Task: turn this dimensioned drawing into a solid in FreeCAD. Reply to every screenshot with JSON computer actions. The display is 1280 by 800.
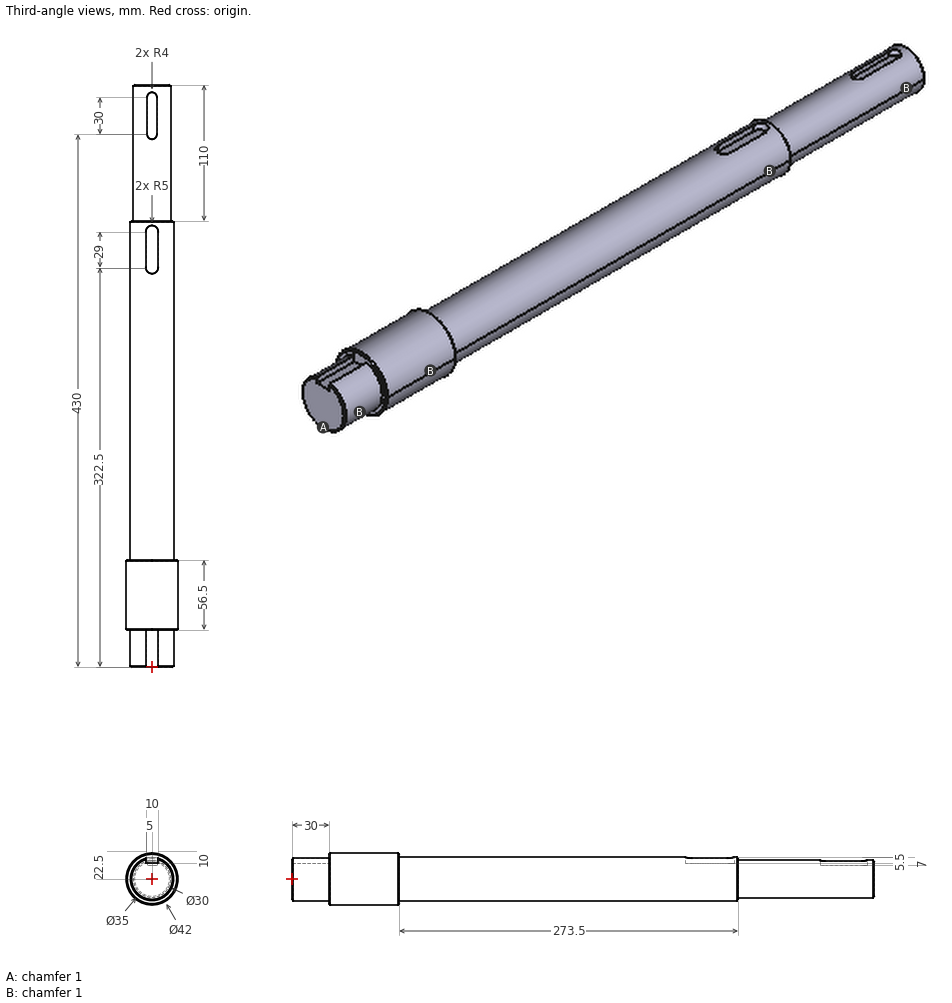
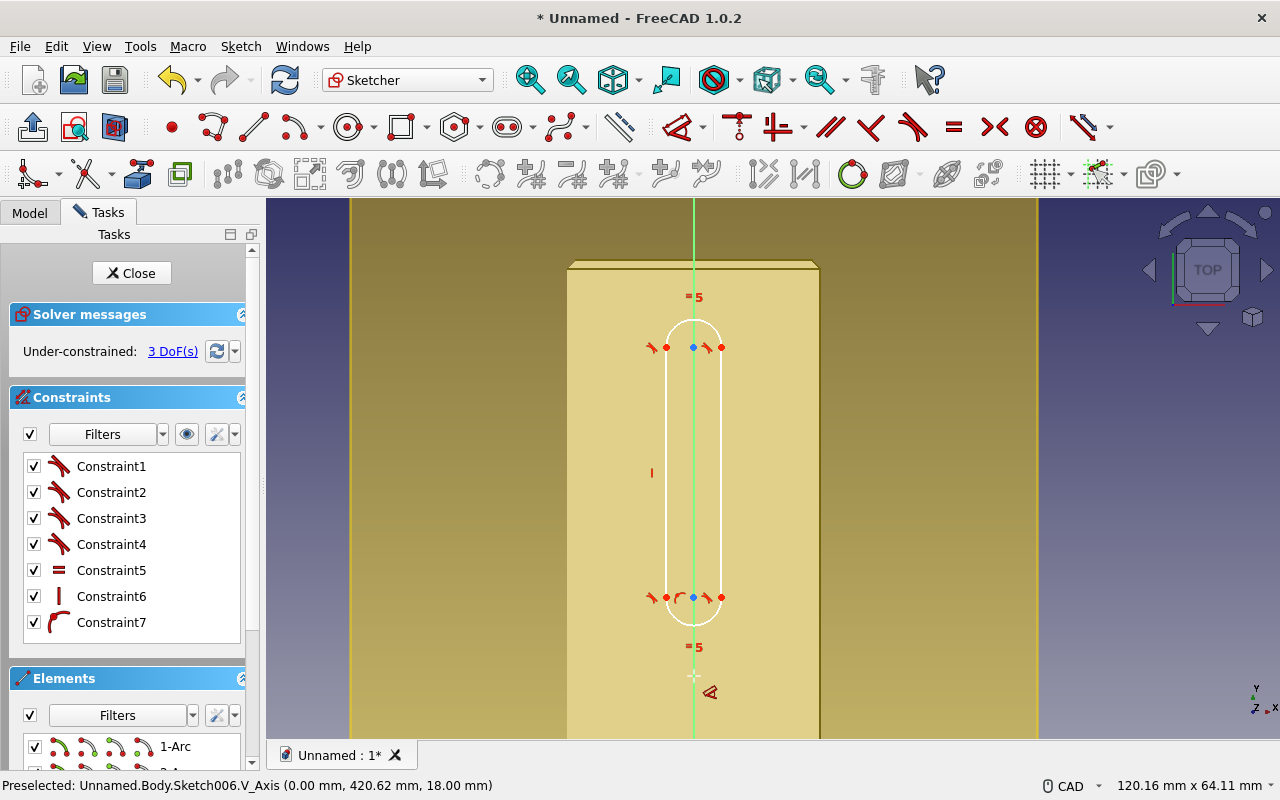
{"action": "left_click", "coordinate": [678, 620]}
{"action": "left_click", "coordinate": [659, 646]}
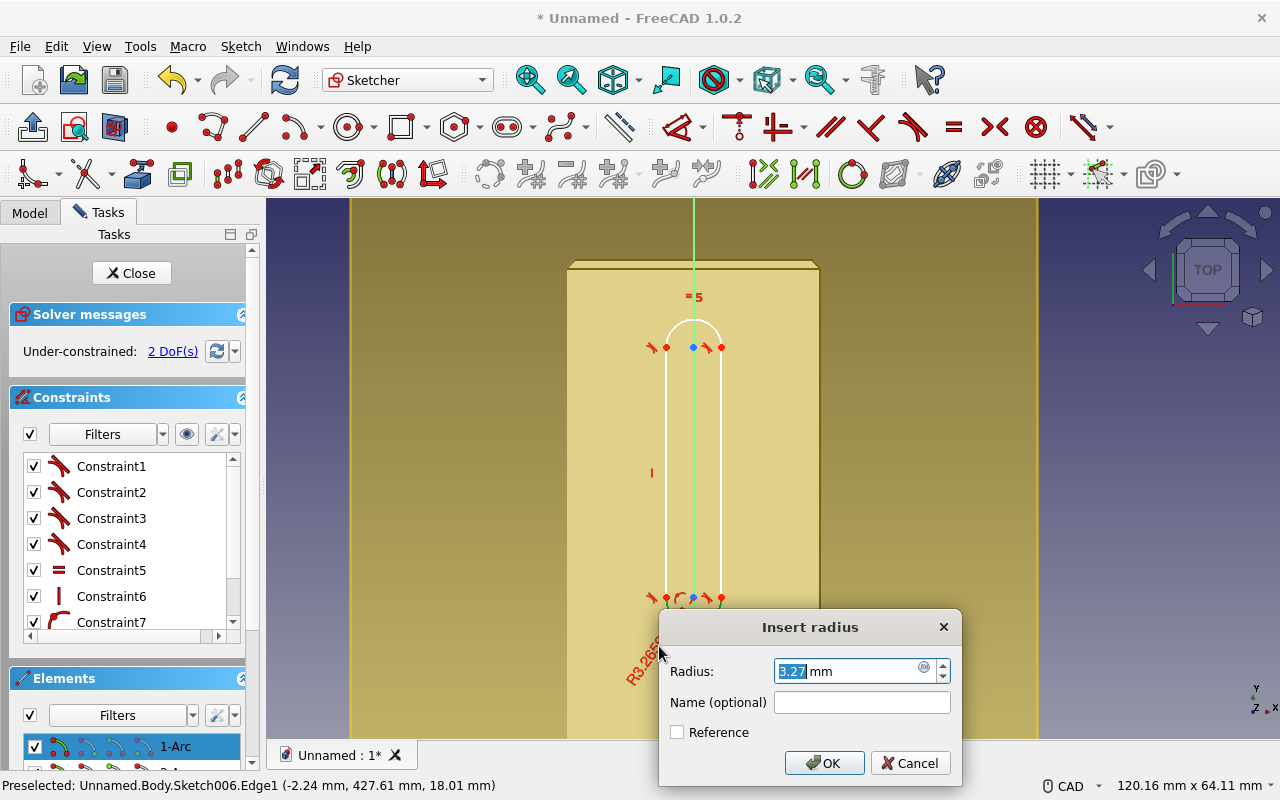
{"action": "type", "text": "4"}
{"action": "key", "text": "Return"}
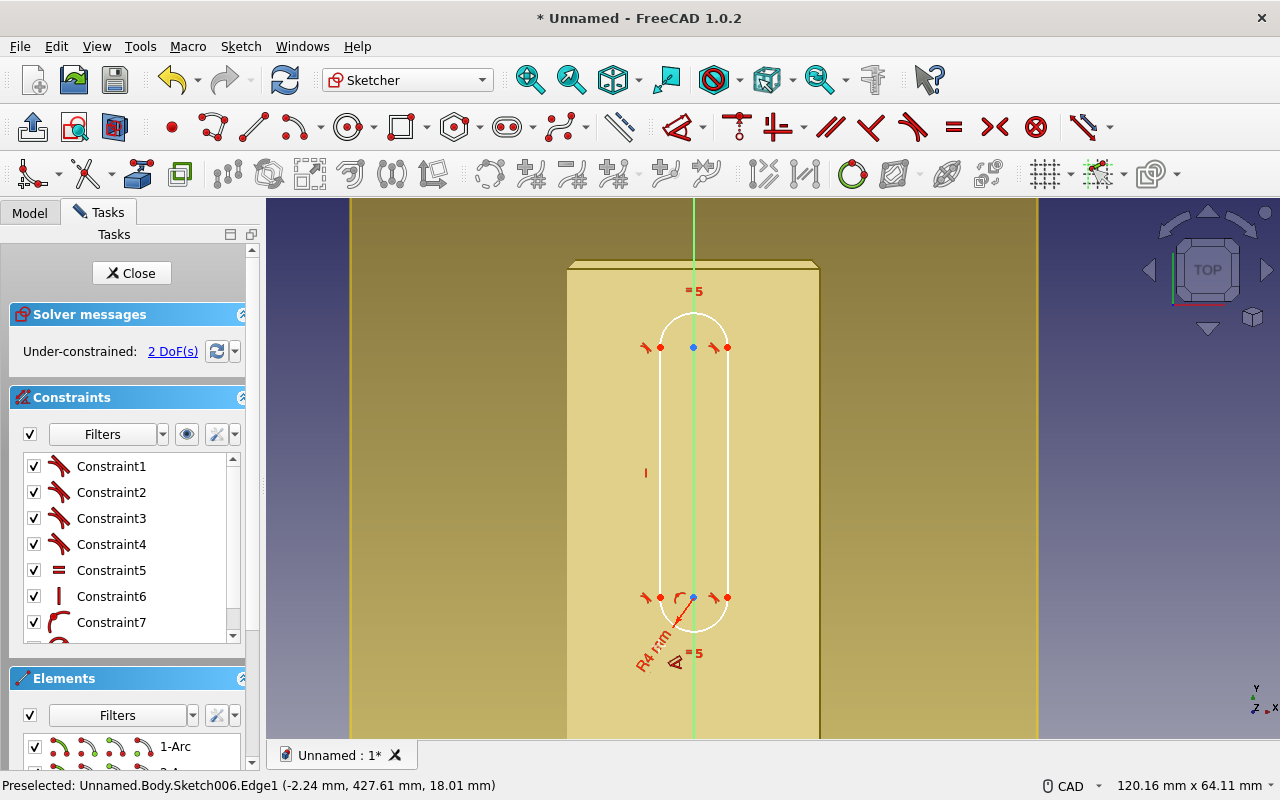
{"action": "left_click", "coordinate": [660, 523]}
{"action": "left_click", "coordinate": [626, 473]}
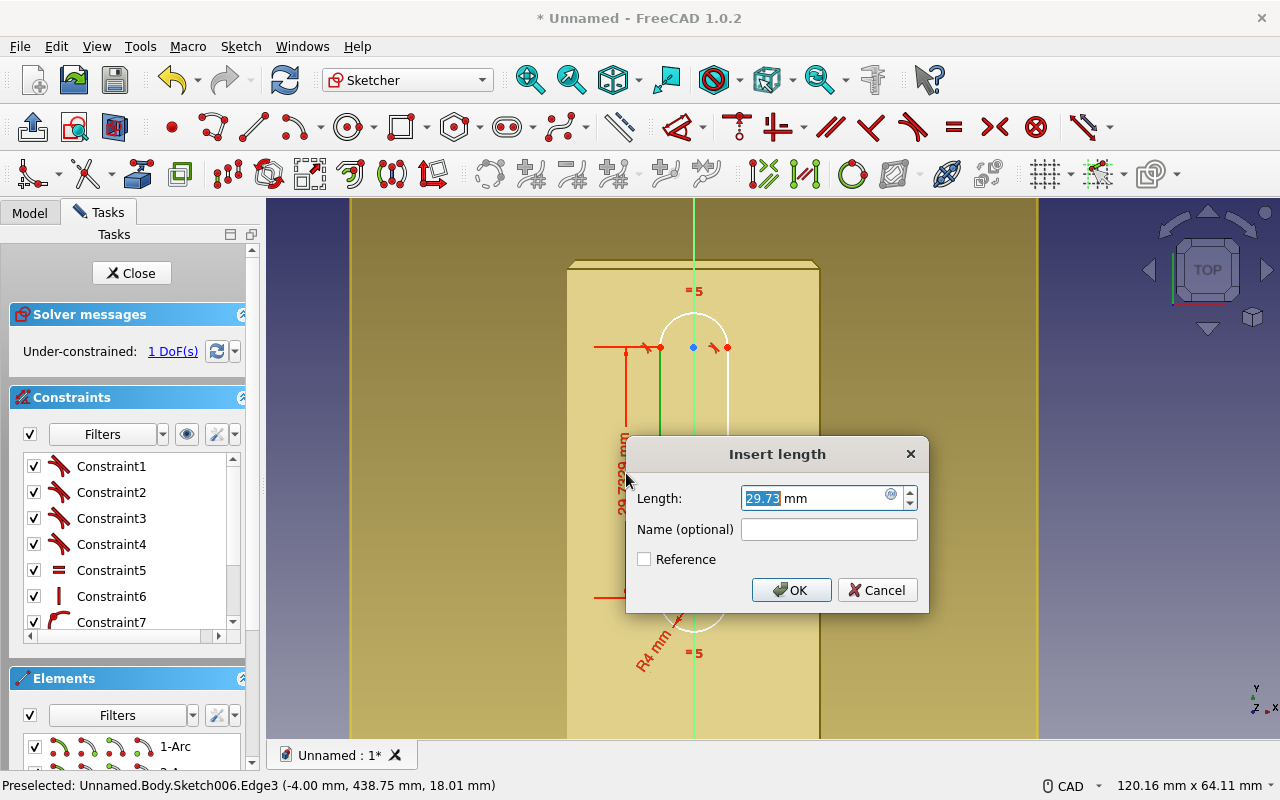
{"action": "type", "text": "30"}
{"action": "key", "text": "Return"}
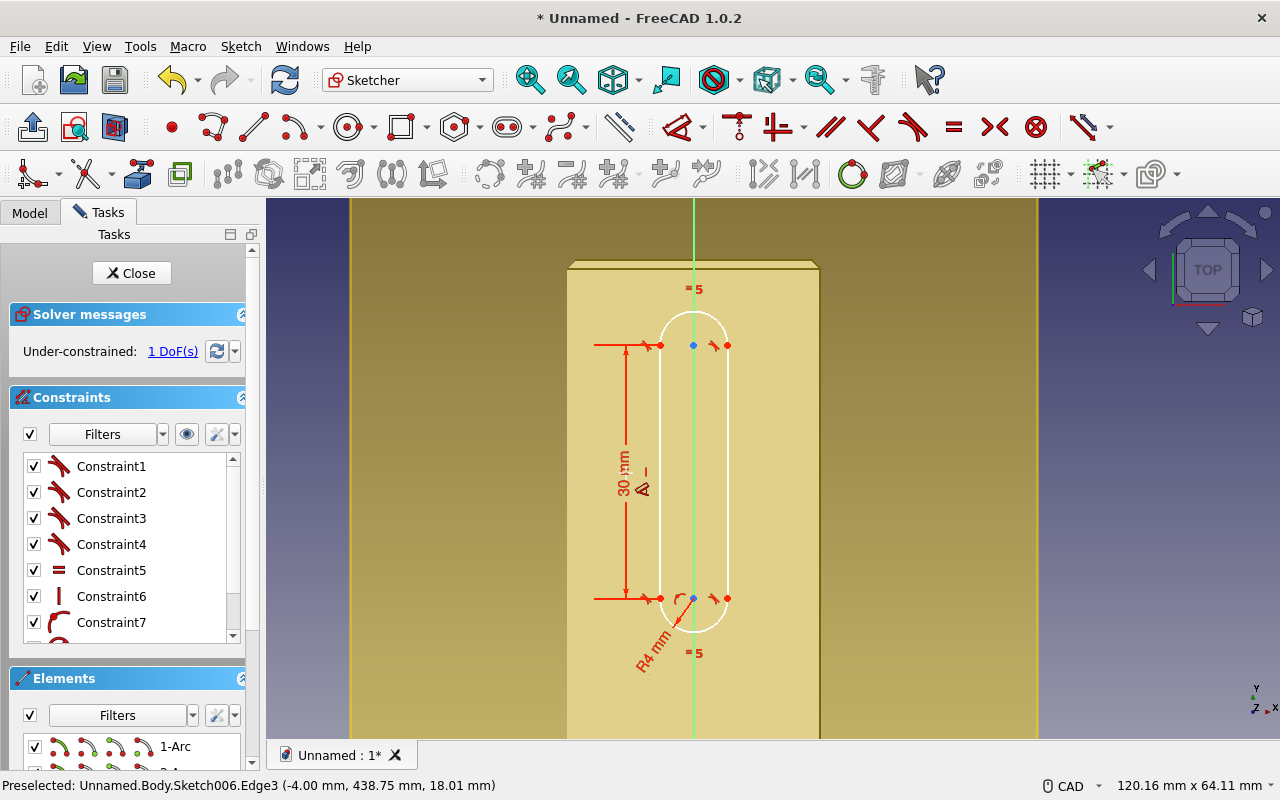
{"action": "left_click", "coordinate": [660, 599]}
{"action": "left_click", "coordinate": [626, 681]}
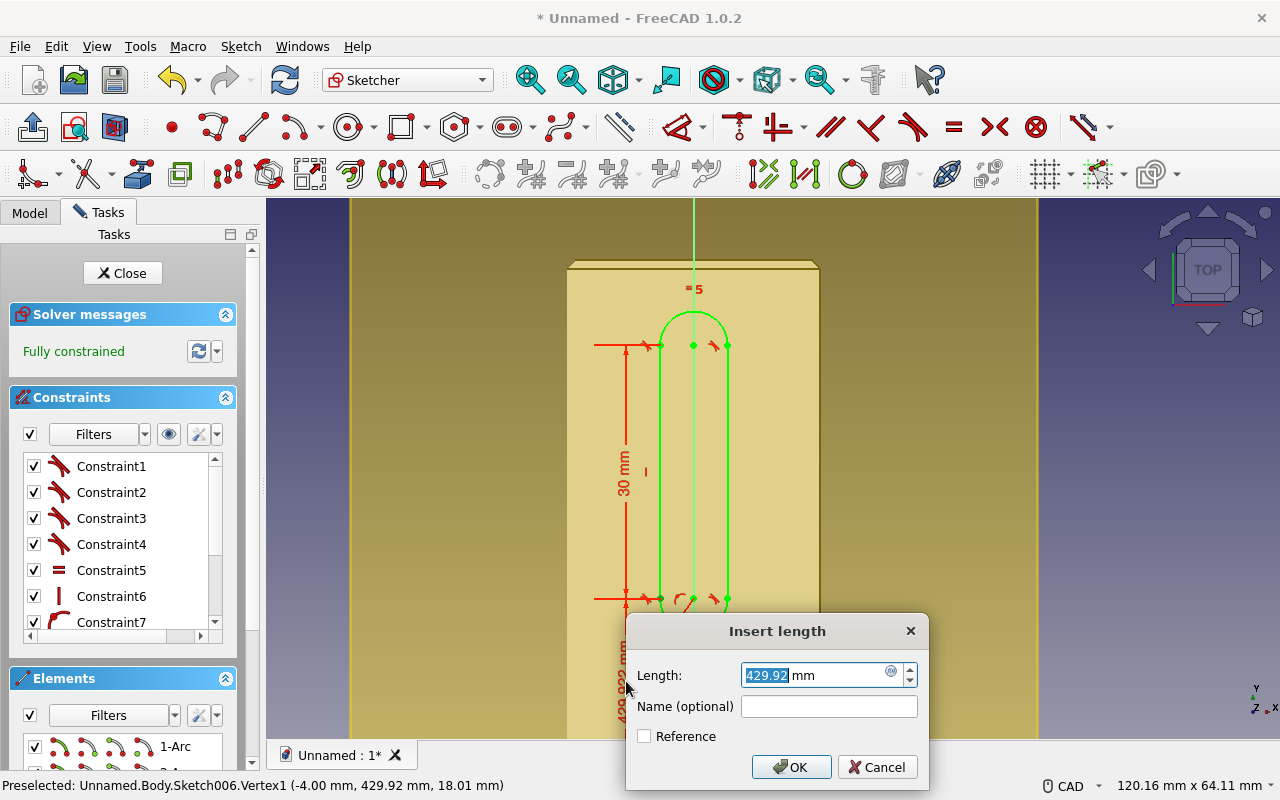
{"action": "type", "text": "430"}
{"action": "key", "text": "Return"}
{"action": "key", "text": "Escape"}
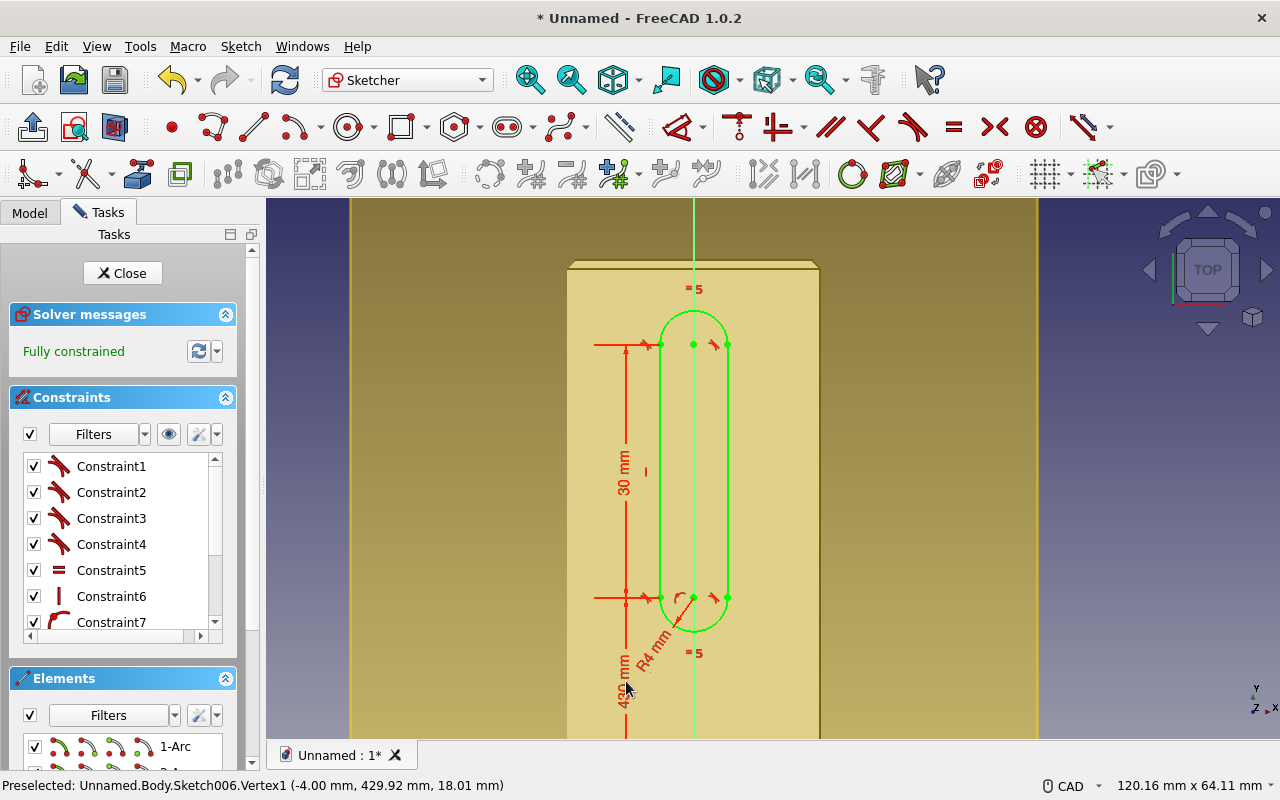
{"action": "left_click", "coordinate": [123, 273]}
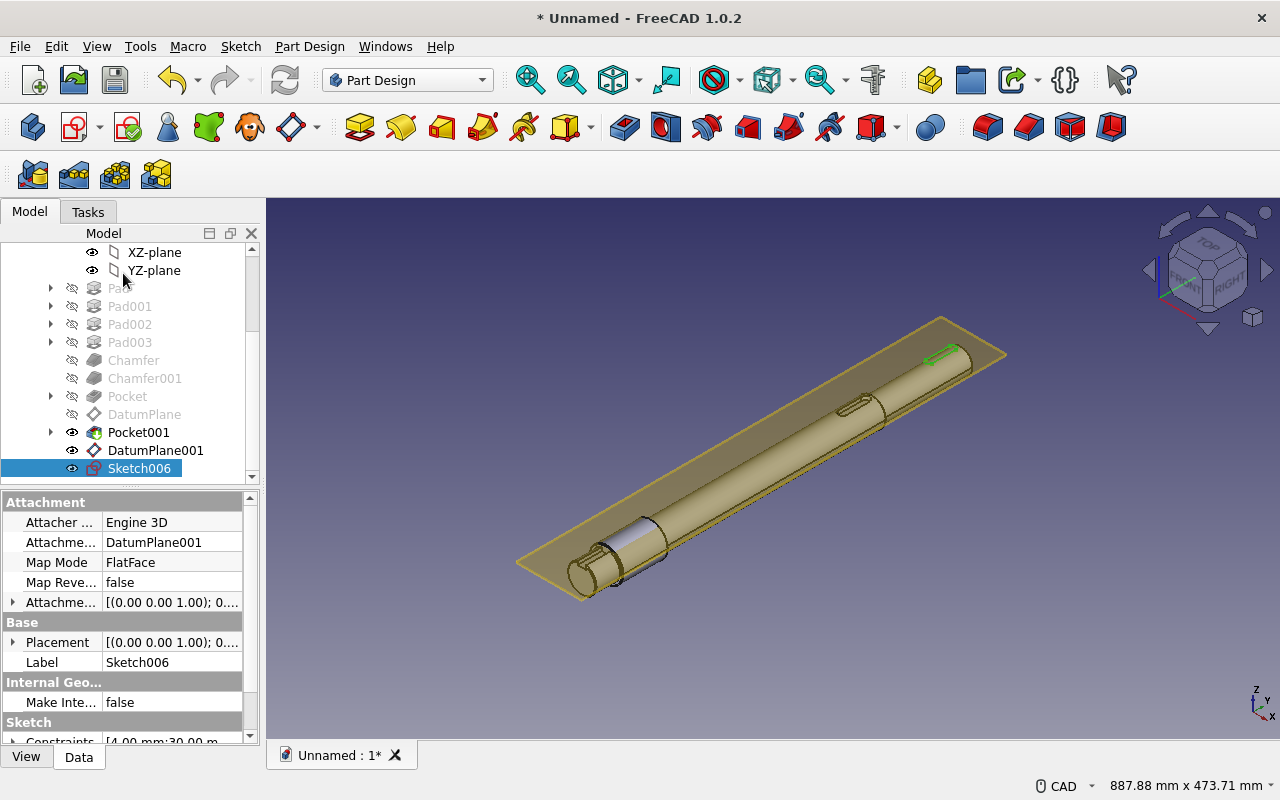
{"action": "left_click", "coordinate": [625, 128]}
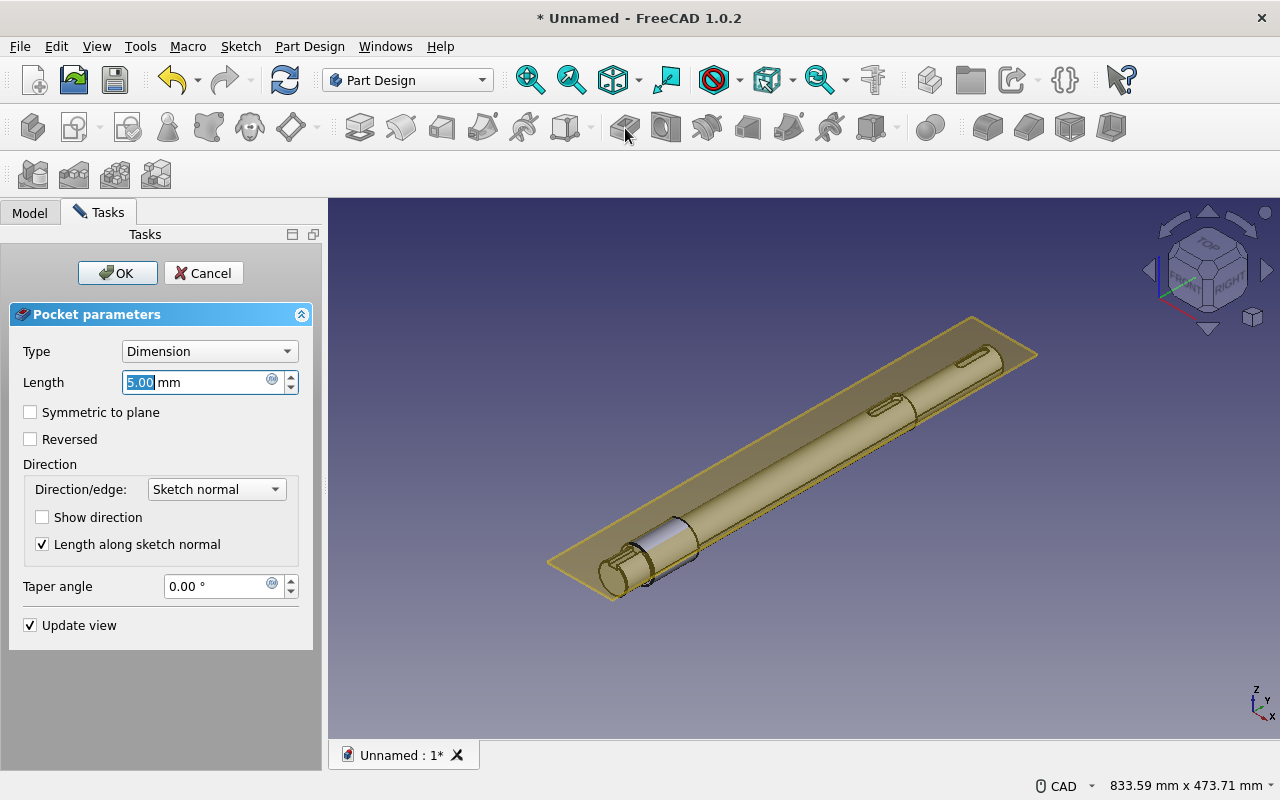
{"action": "type", "text": "7"}
{"action": "key", "text": "Tab"}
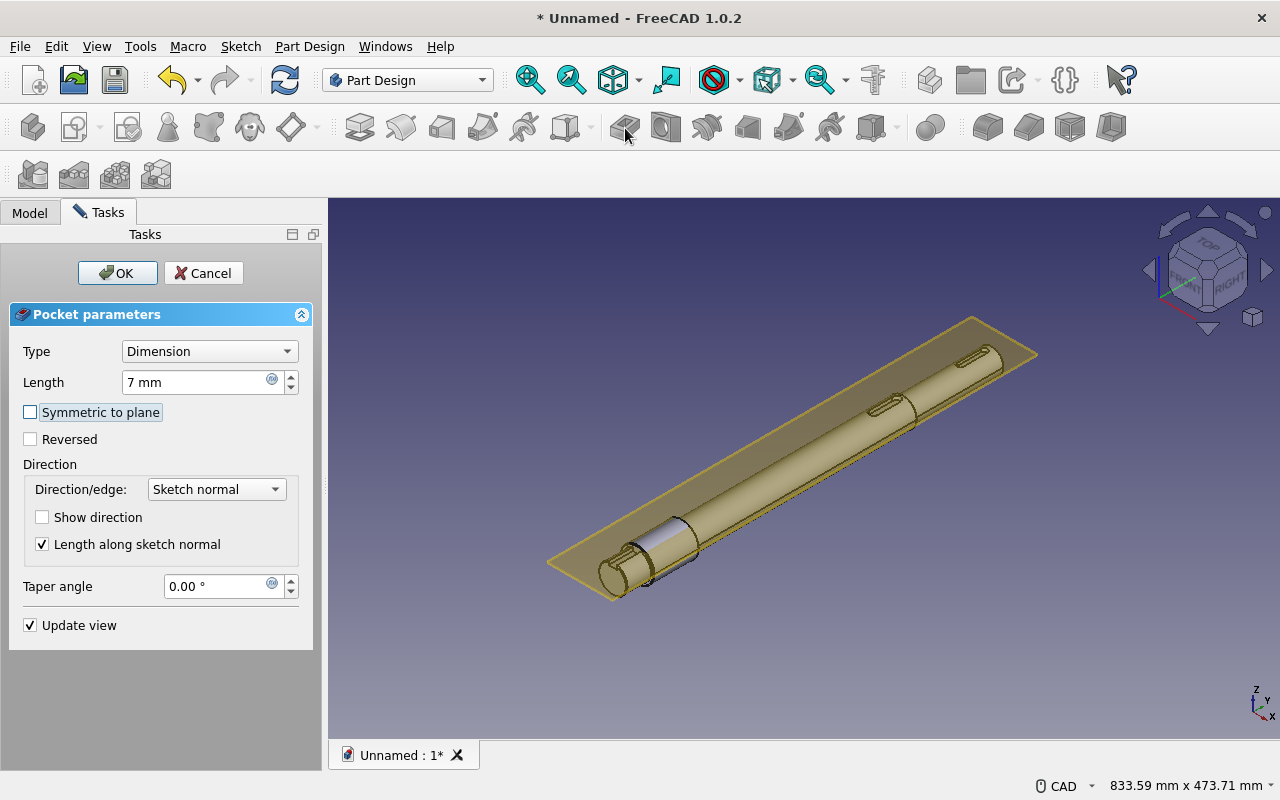
{"action": "left_click", "coordinate": [118, 273]}